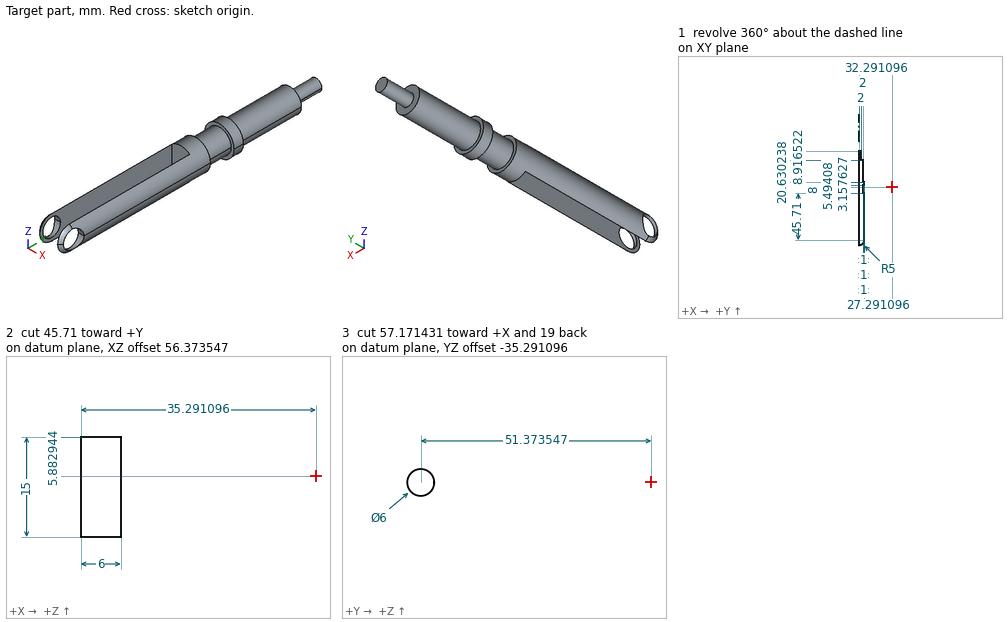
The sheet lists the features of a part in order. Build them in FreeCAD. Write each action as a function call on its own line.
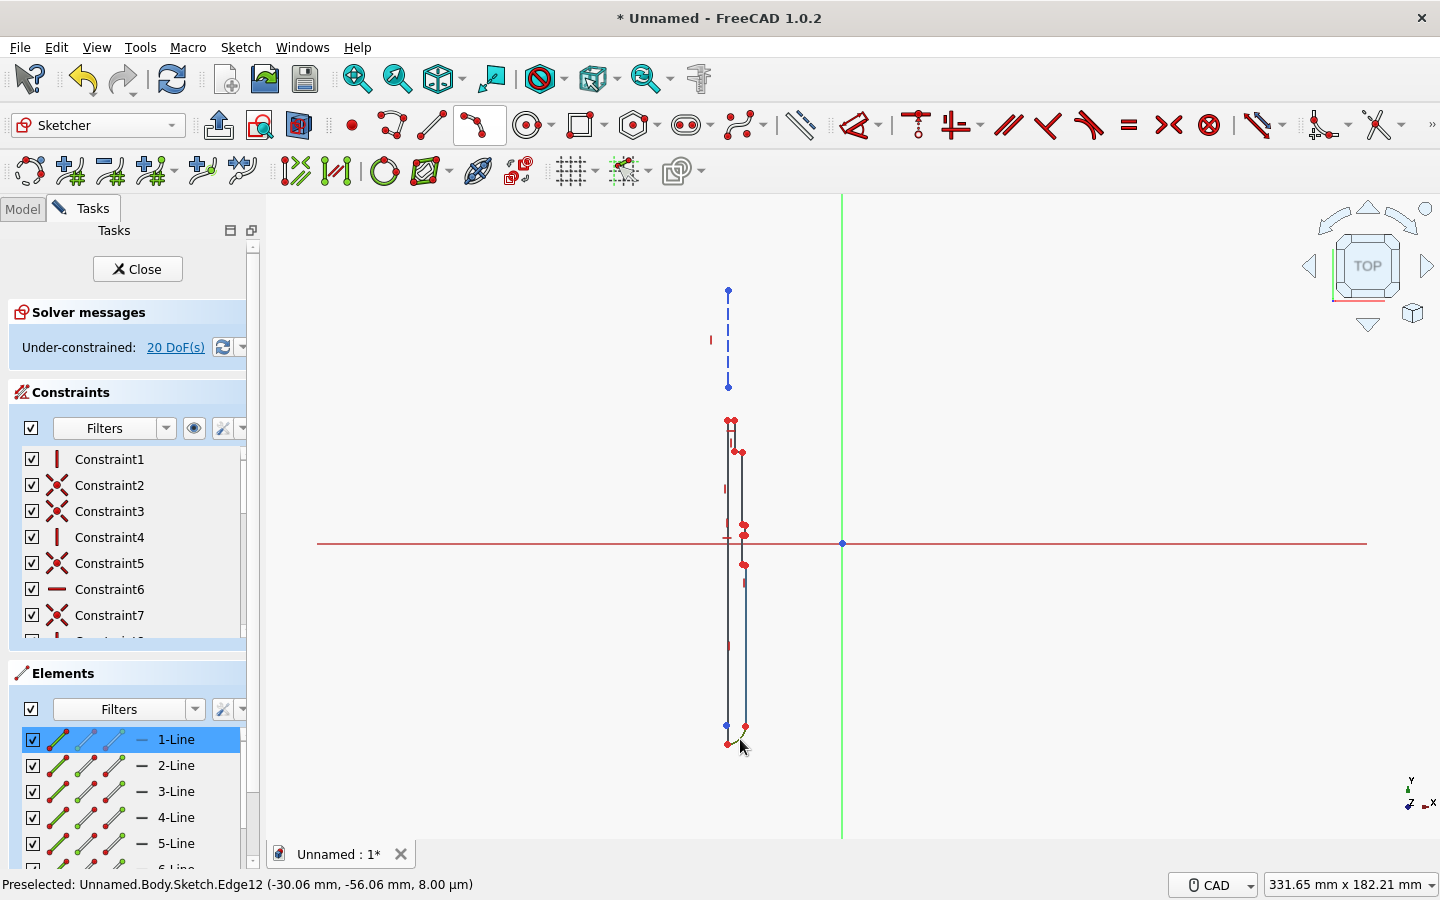
click(1090, 126)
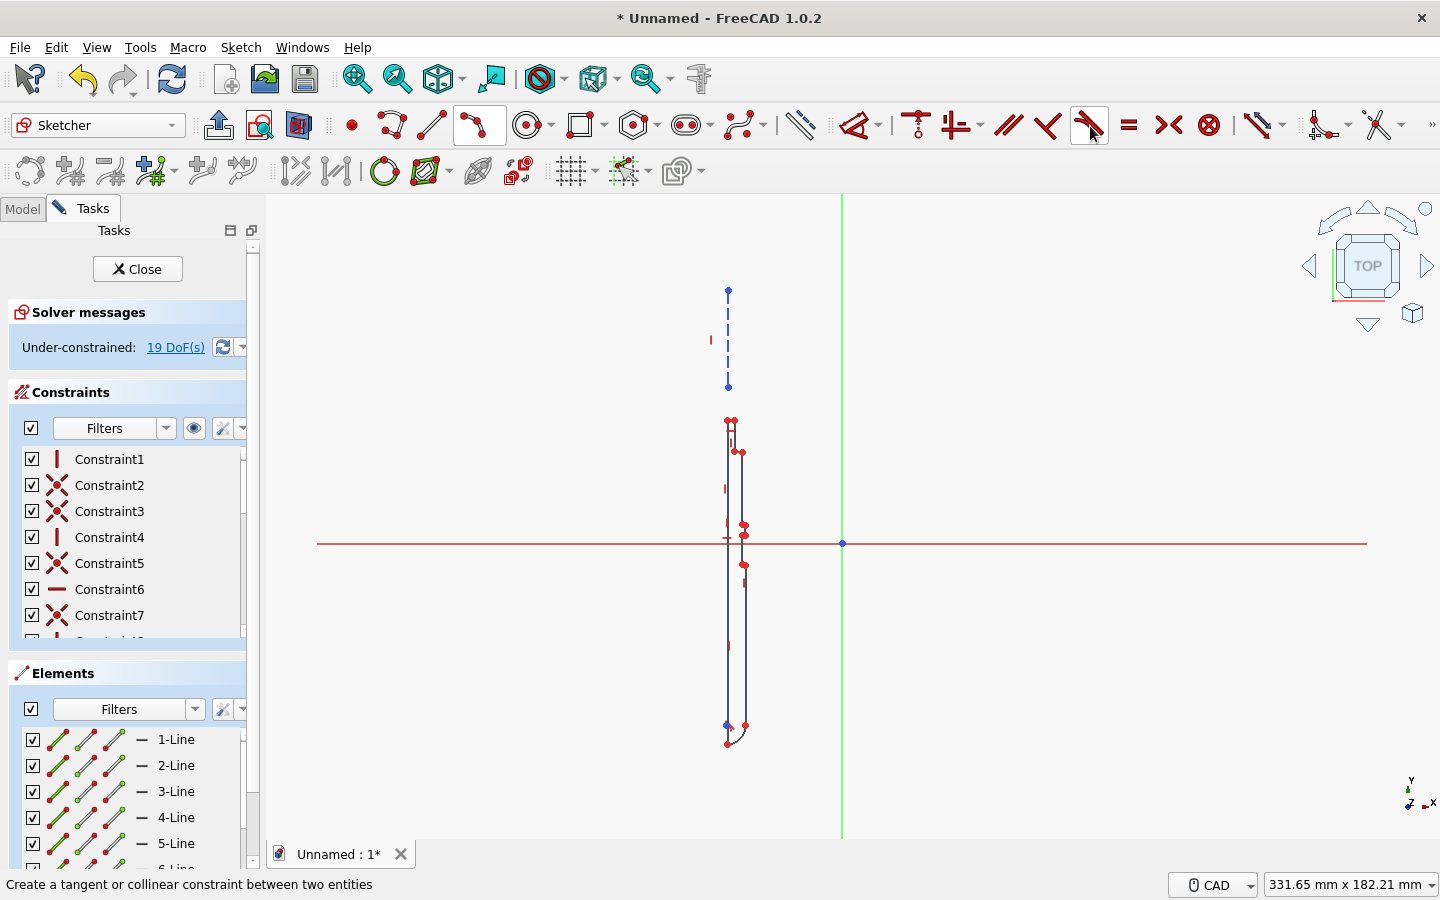
scroll(744, 565, up, 11)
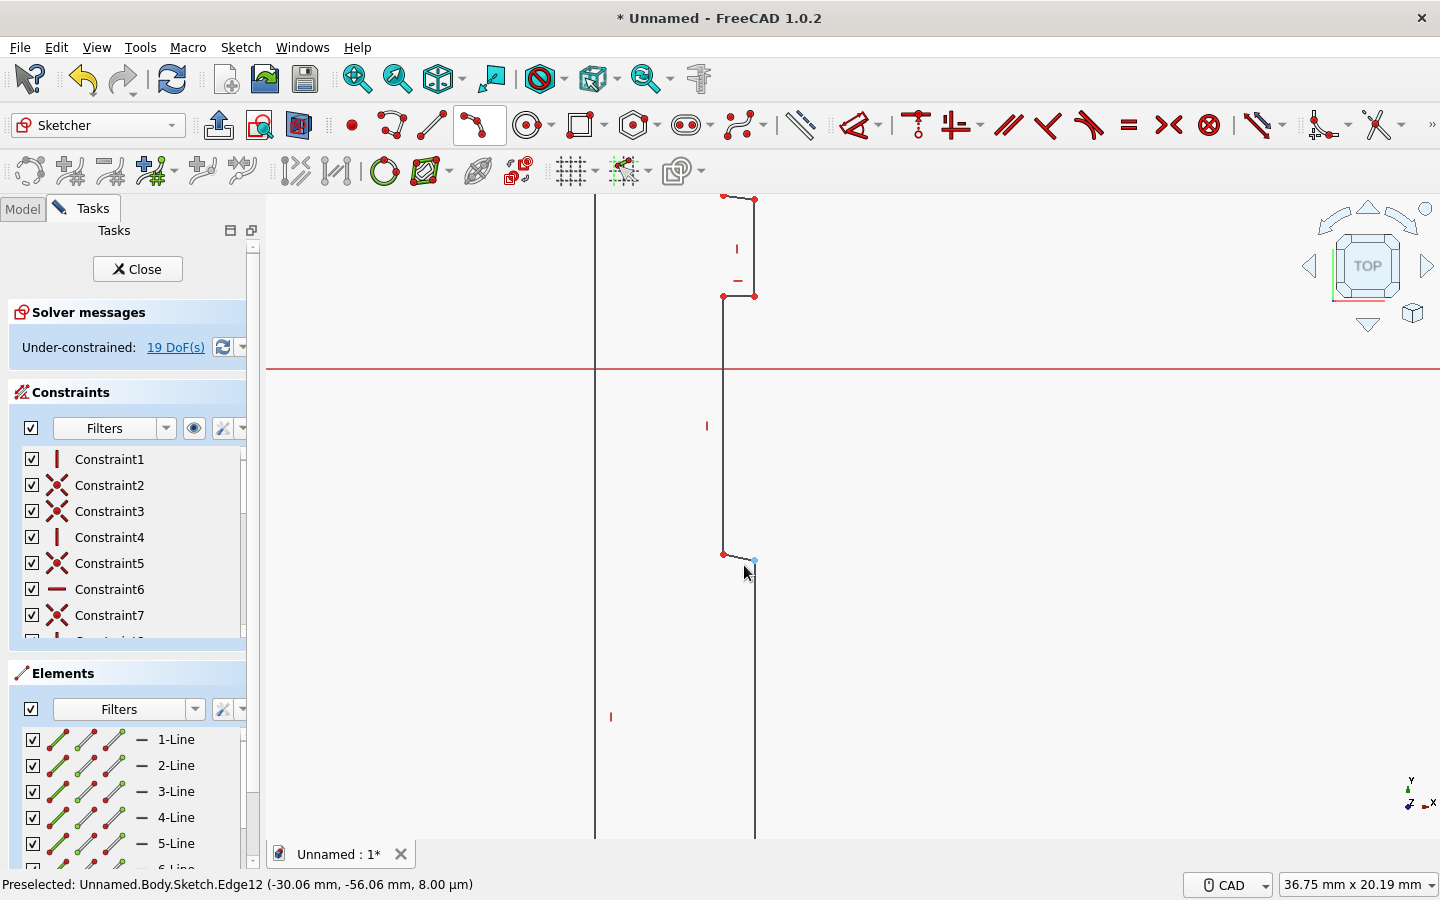
click(739, 558)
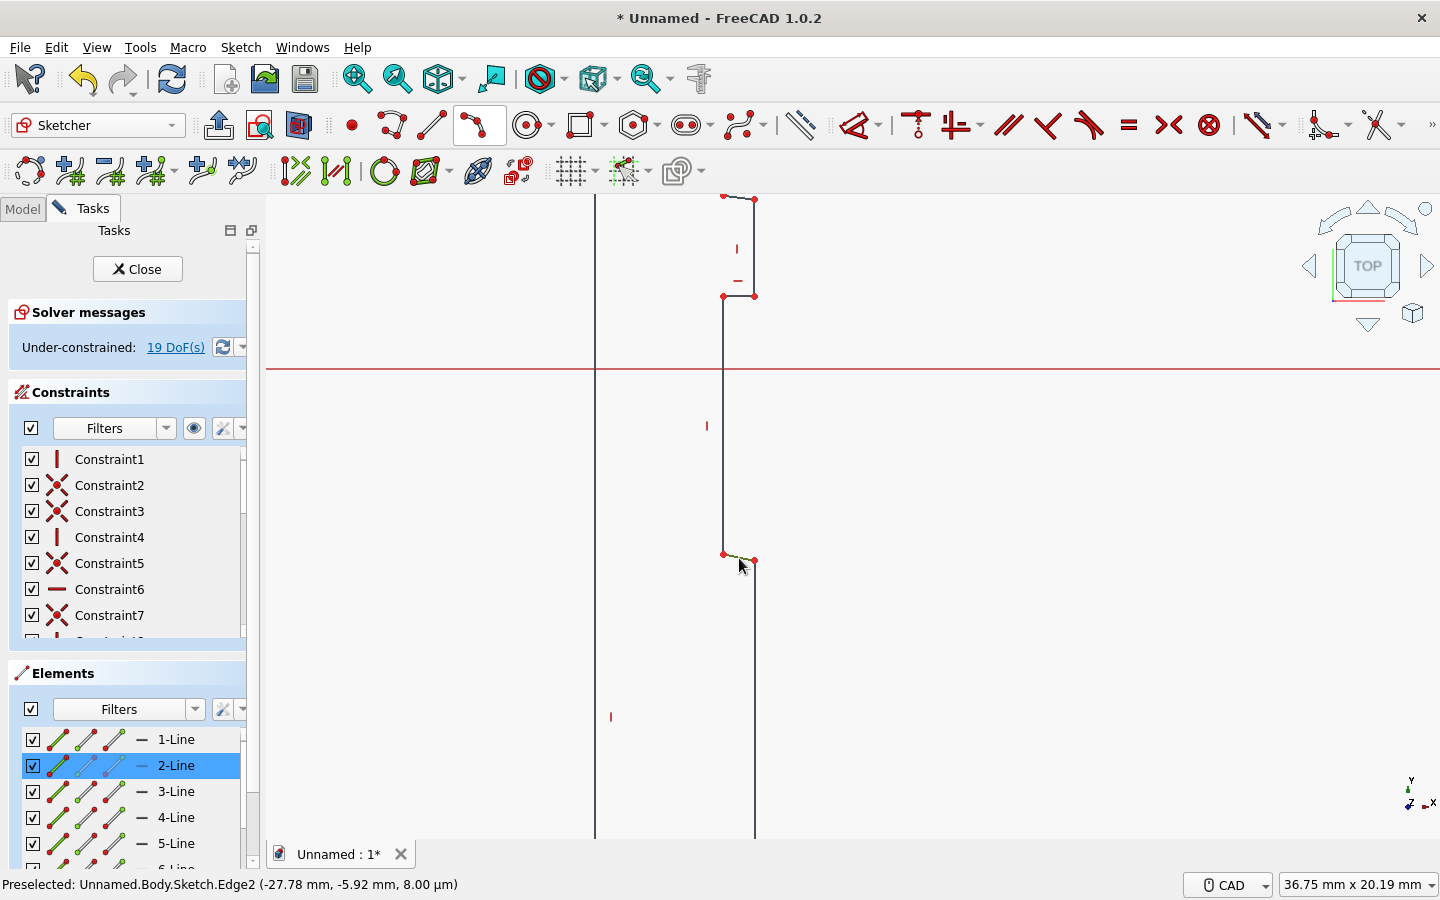
click(982, 126)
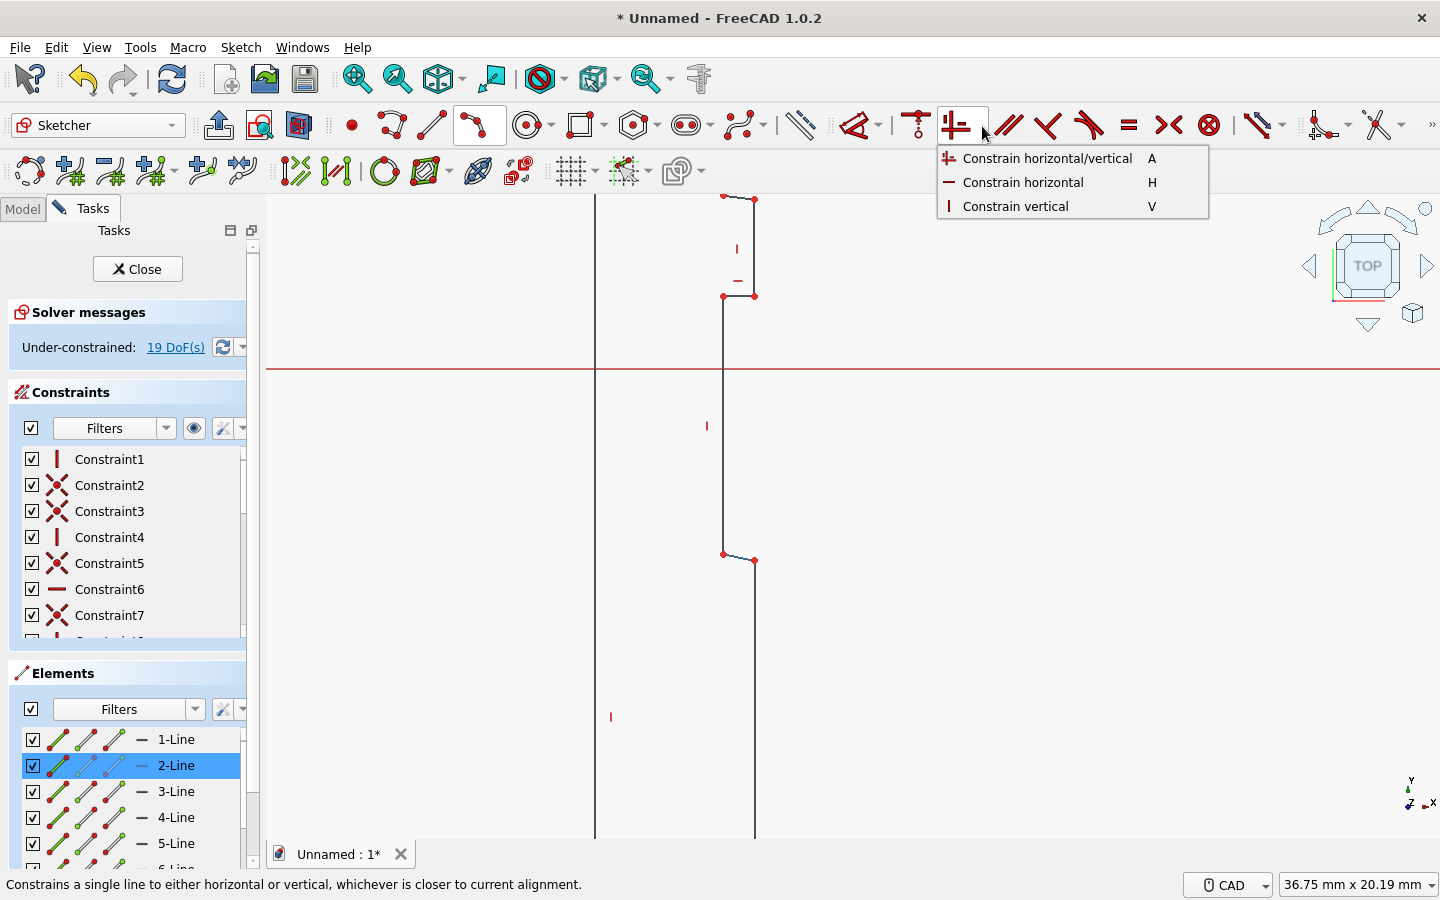
click(1073, 182)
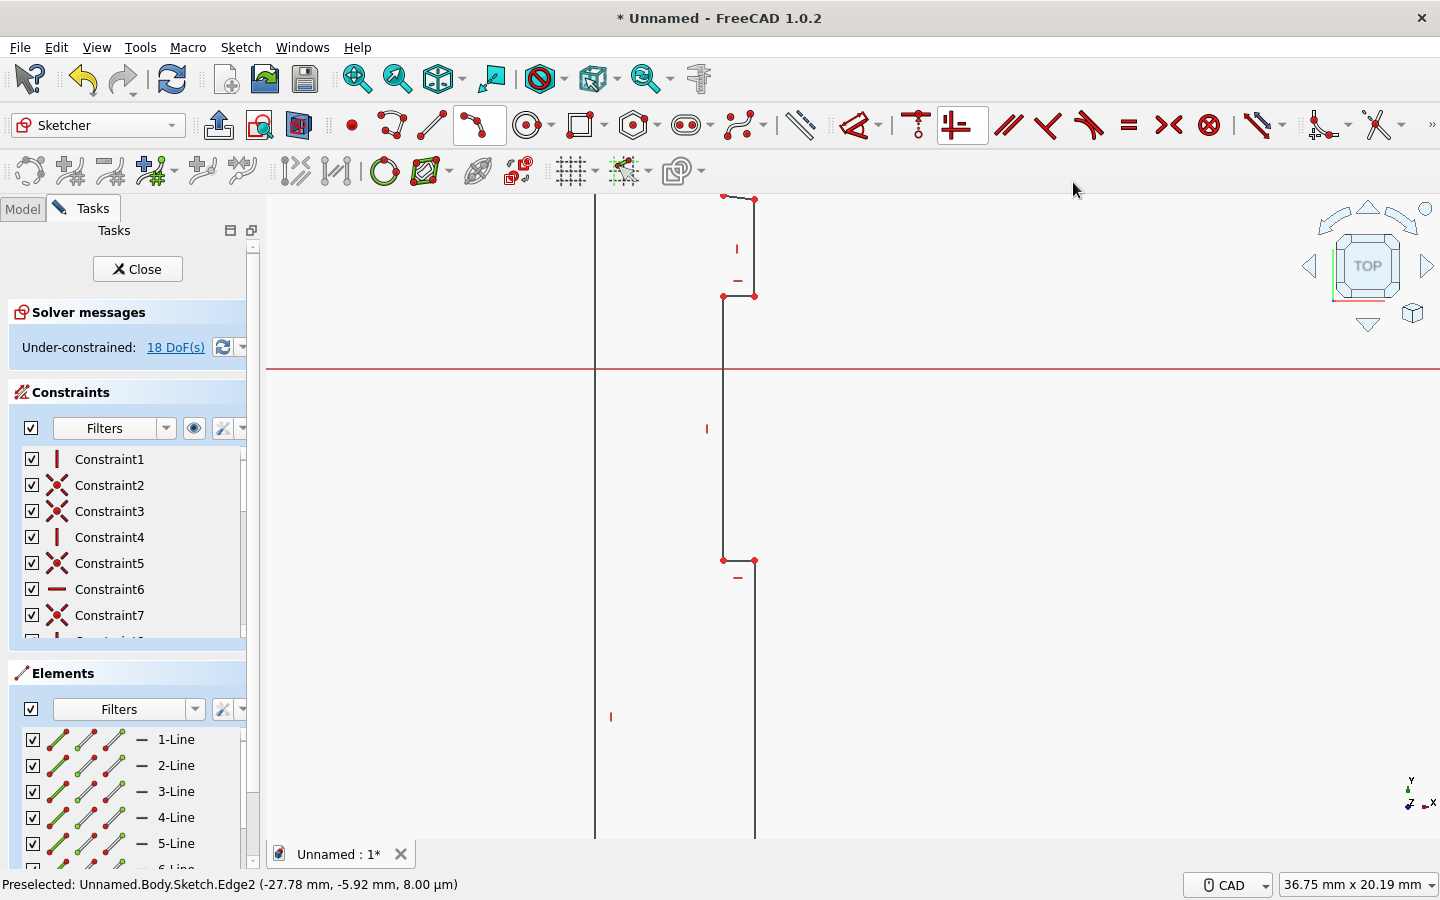
scroll(744, 565, down, 11)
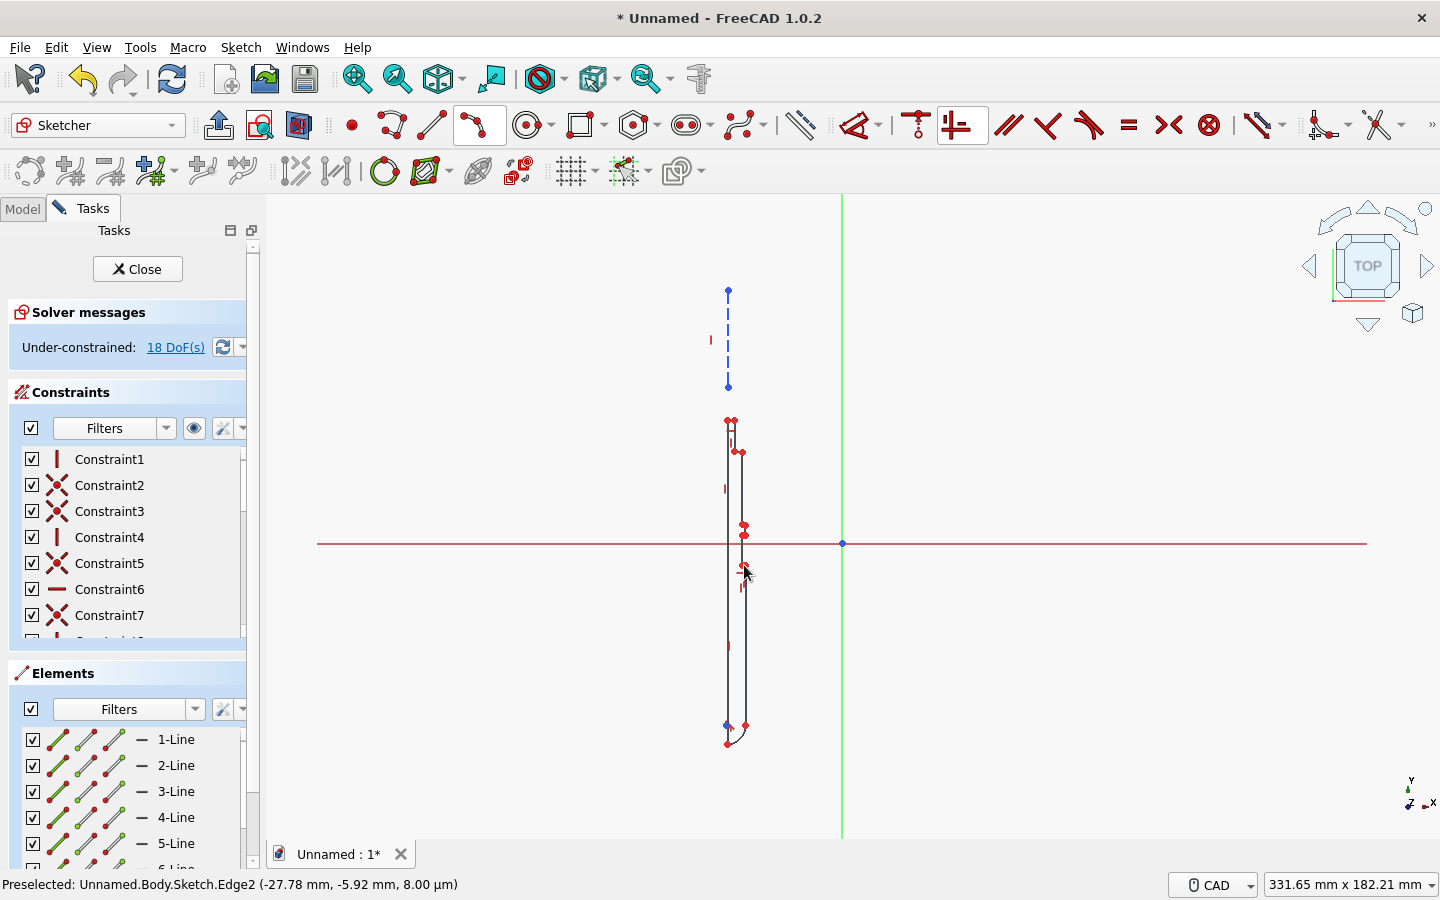
scroll(744, 525, up, 14)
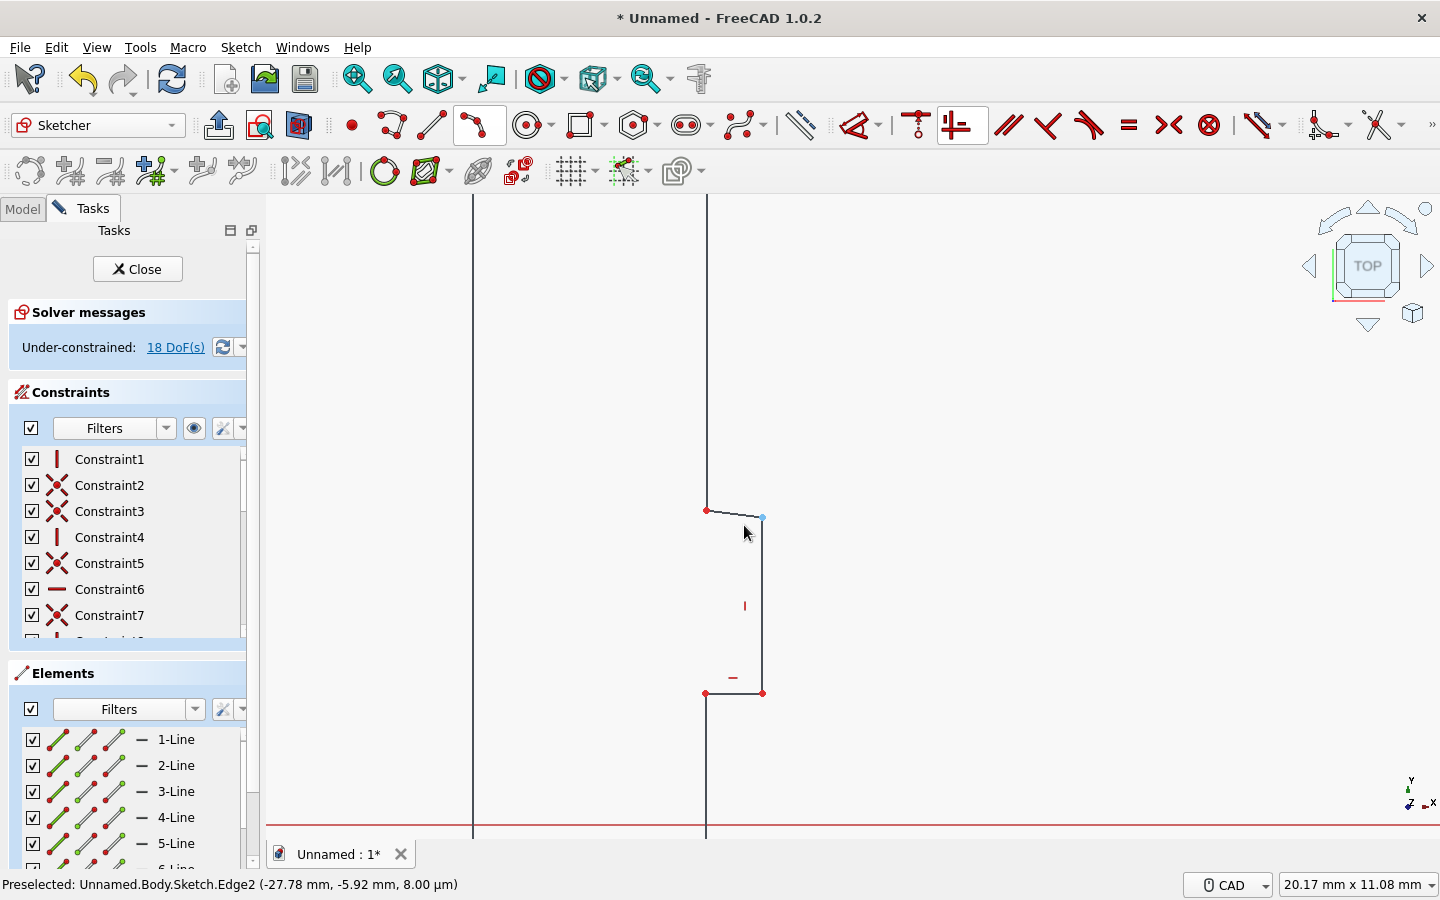
click(745, 515)